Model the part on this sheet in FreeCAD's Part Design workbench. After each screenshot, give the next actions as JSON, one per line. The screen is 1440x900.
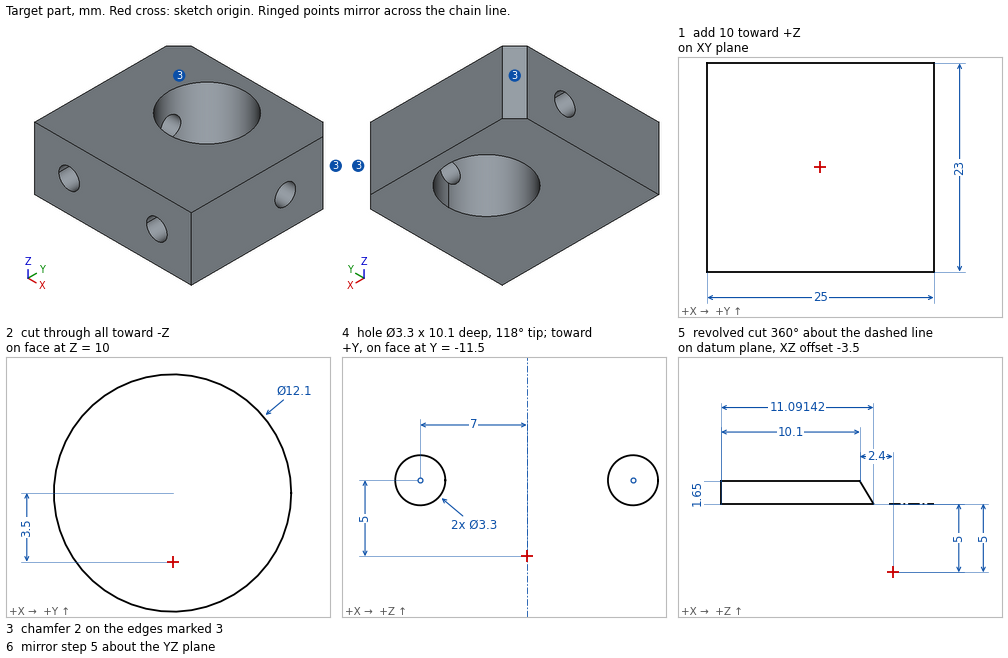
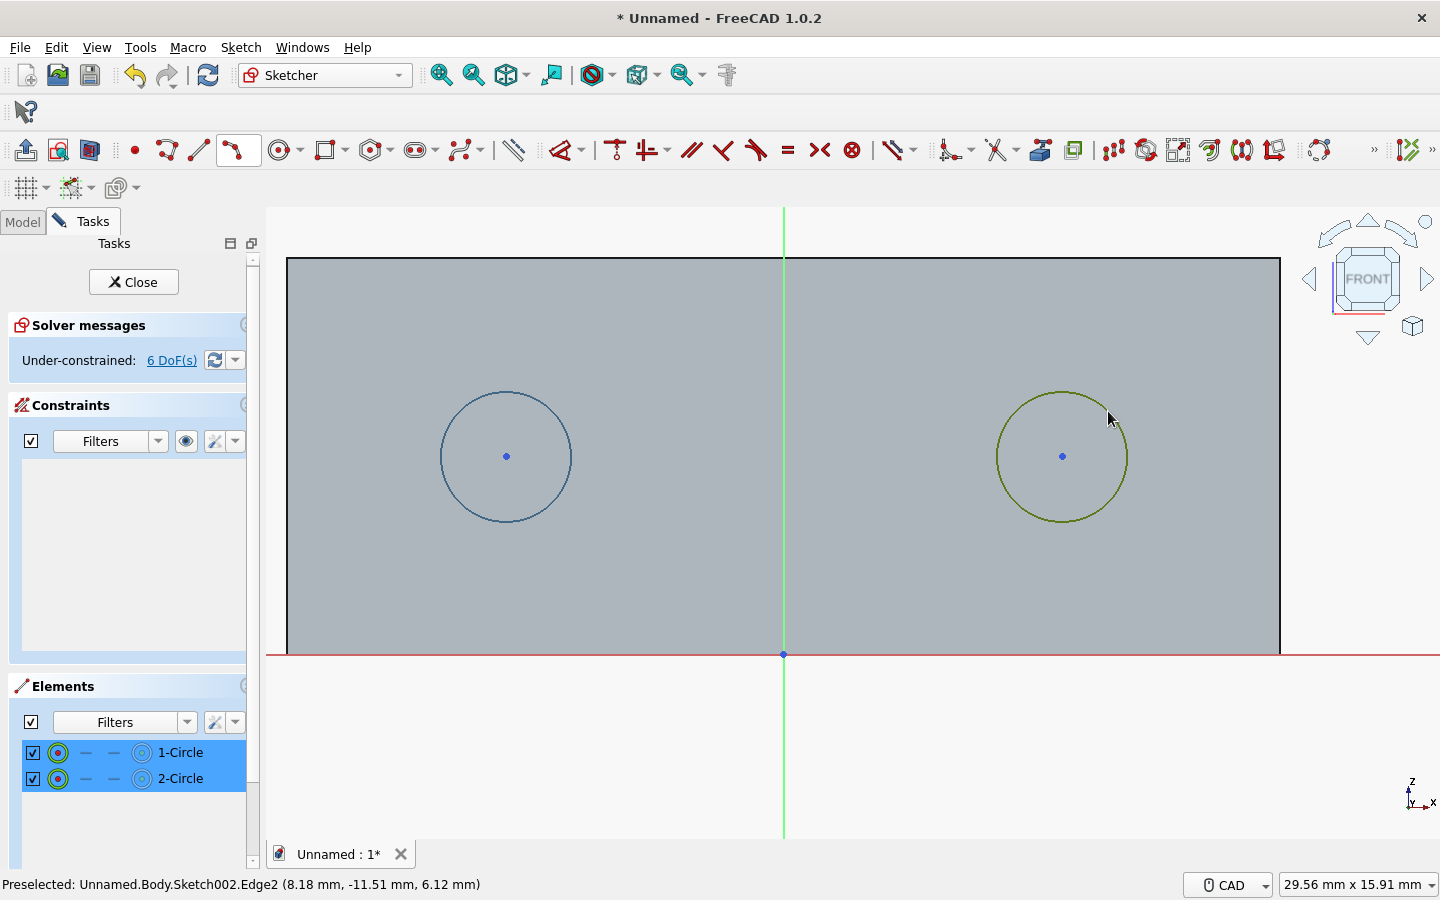
{"action": "left_click", "coordinate": [788, 150]}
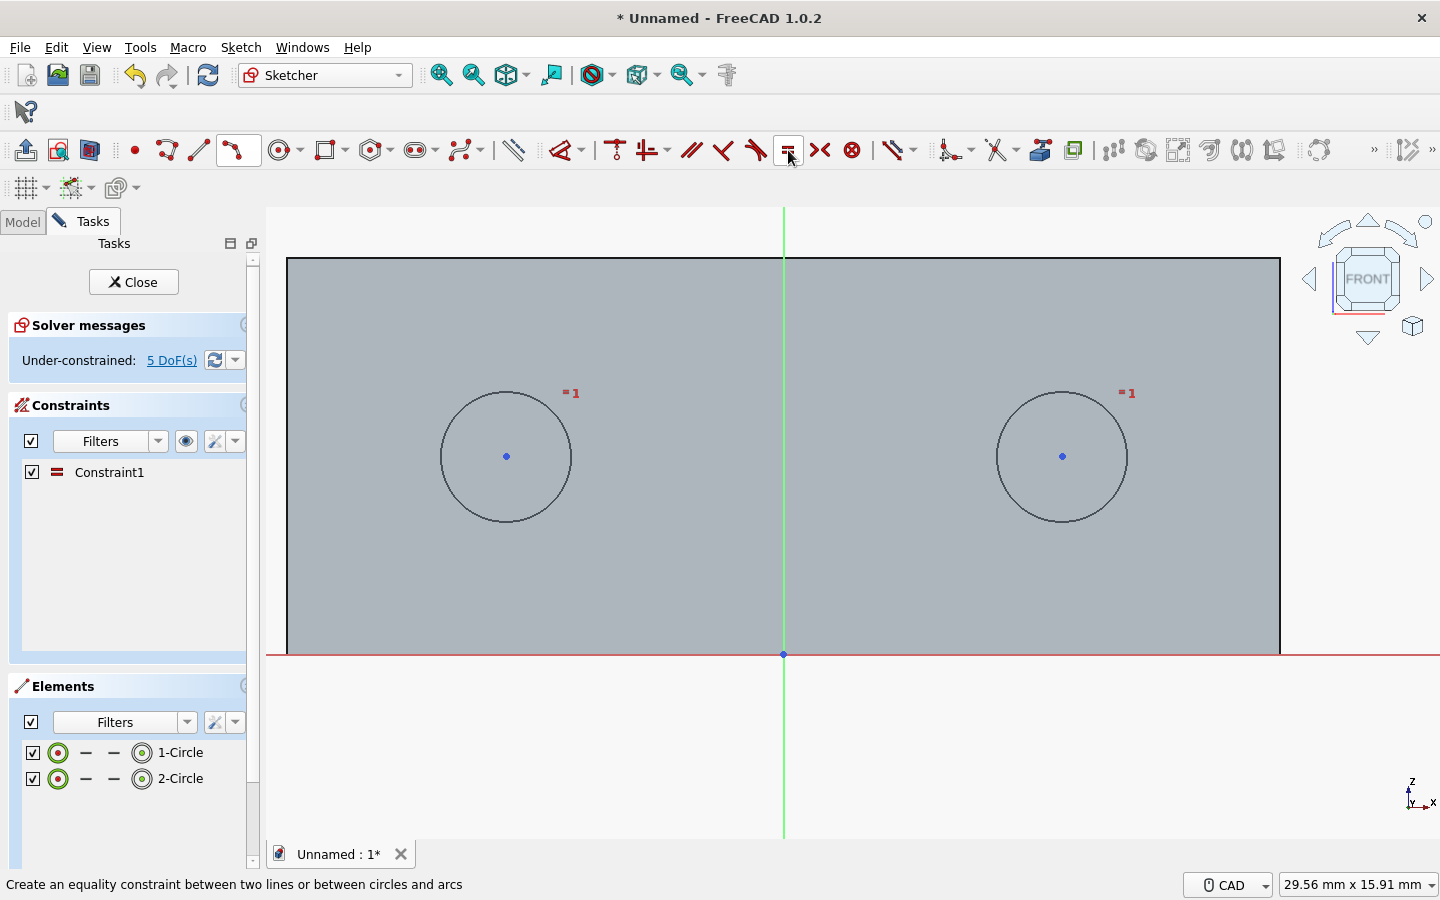
{"action": "left_click", "coordinate": [506, 457]}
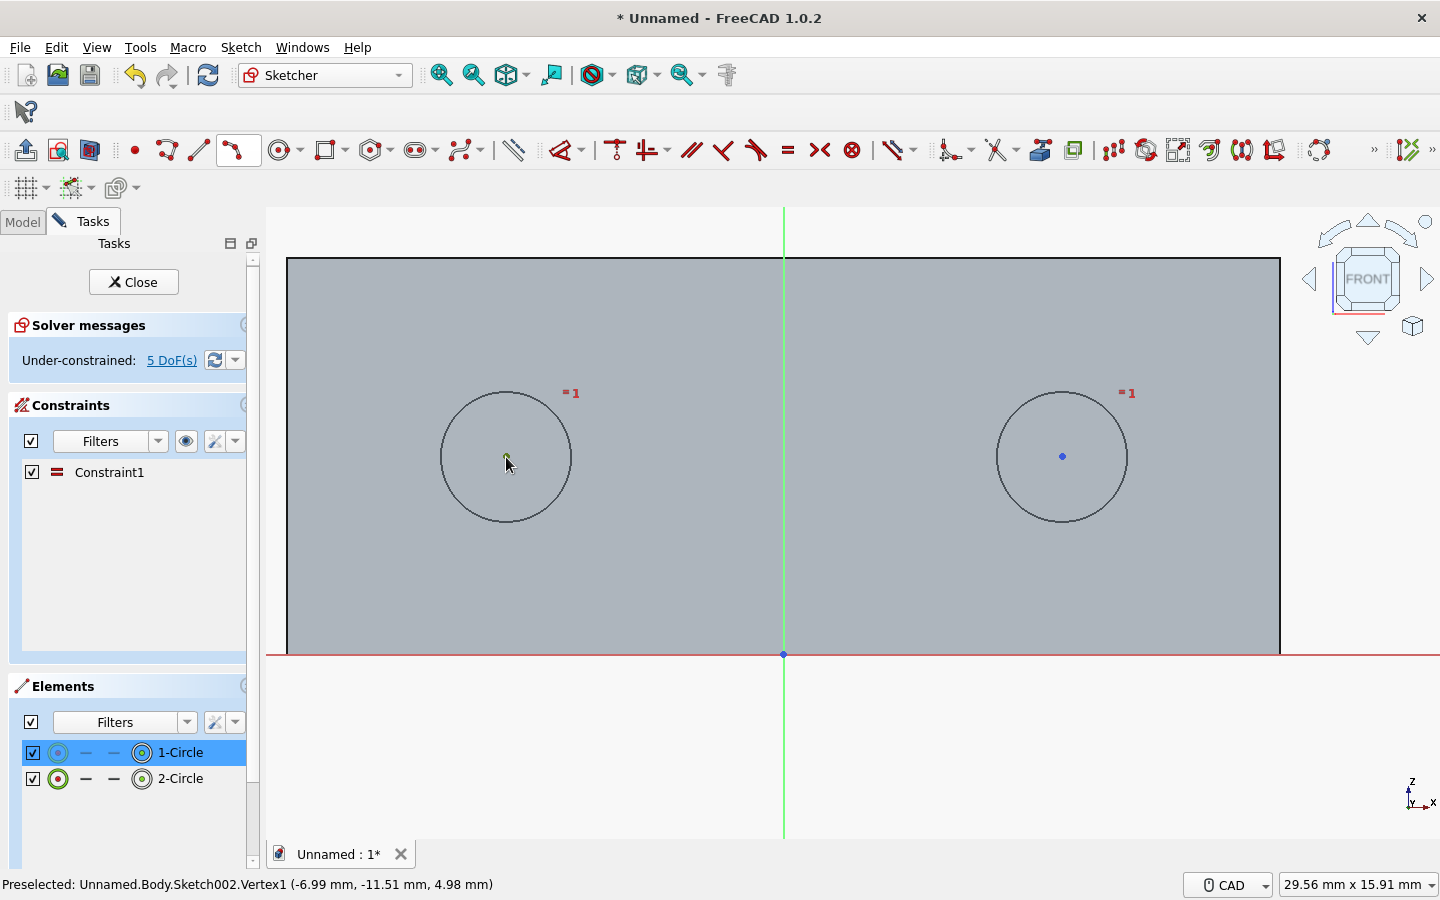
{"action": "left_click", "coordinate": [1062, 457]}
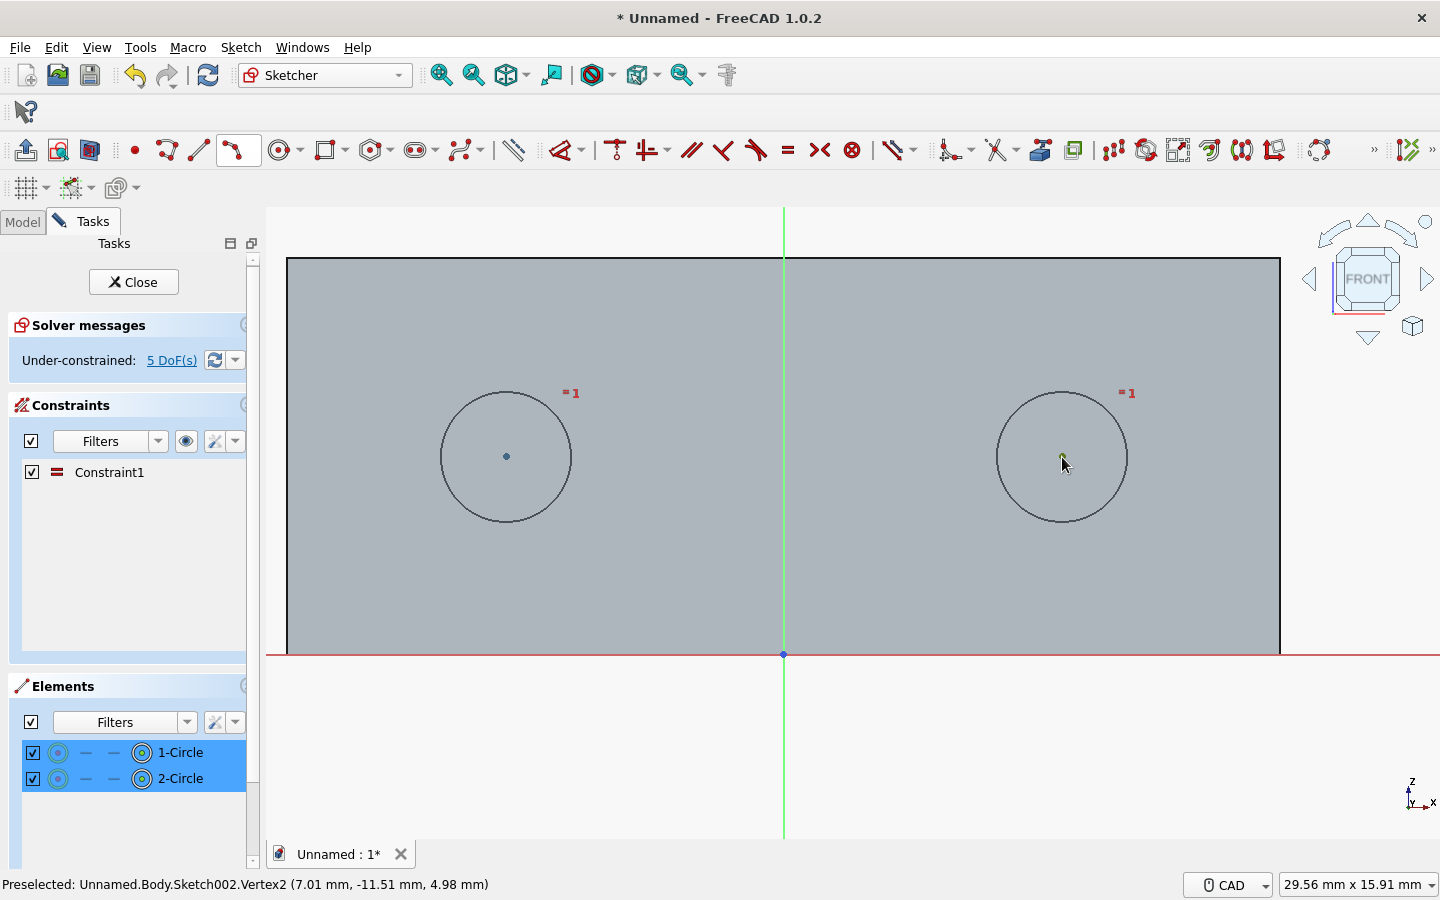
{"action": "left_click", "coordinate": [784, 770]}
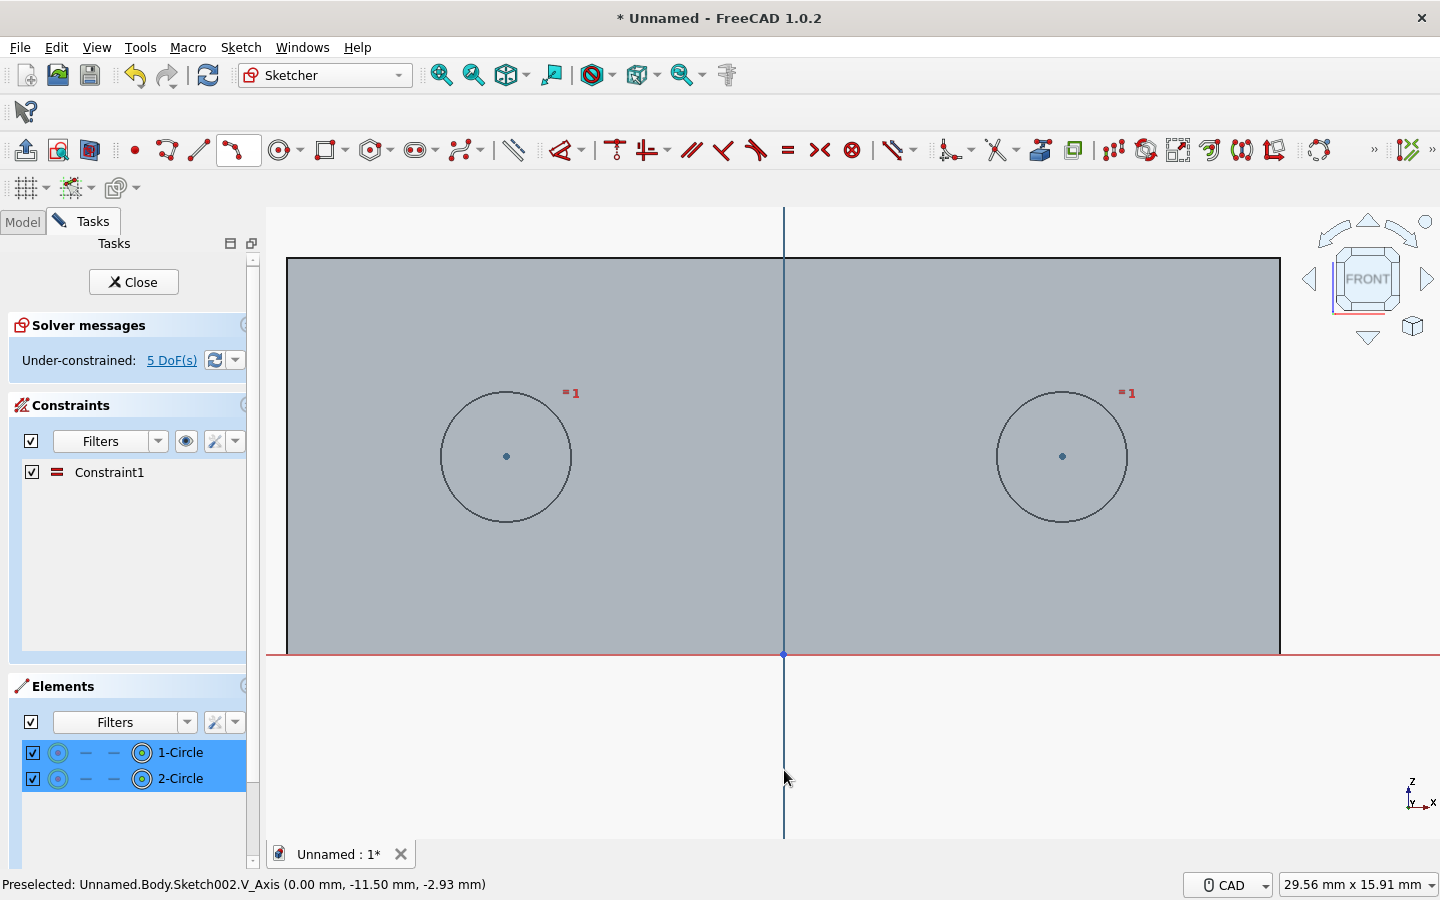
{"action": "key", "text": "s"}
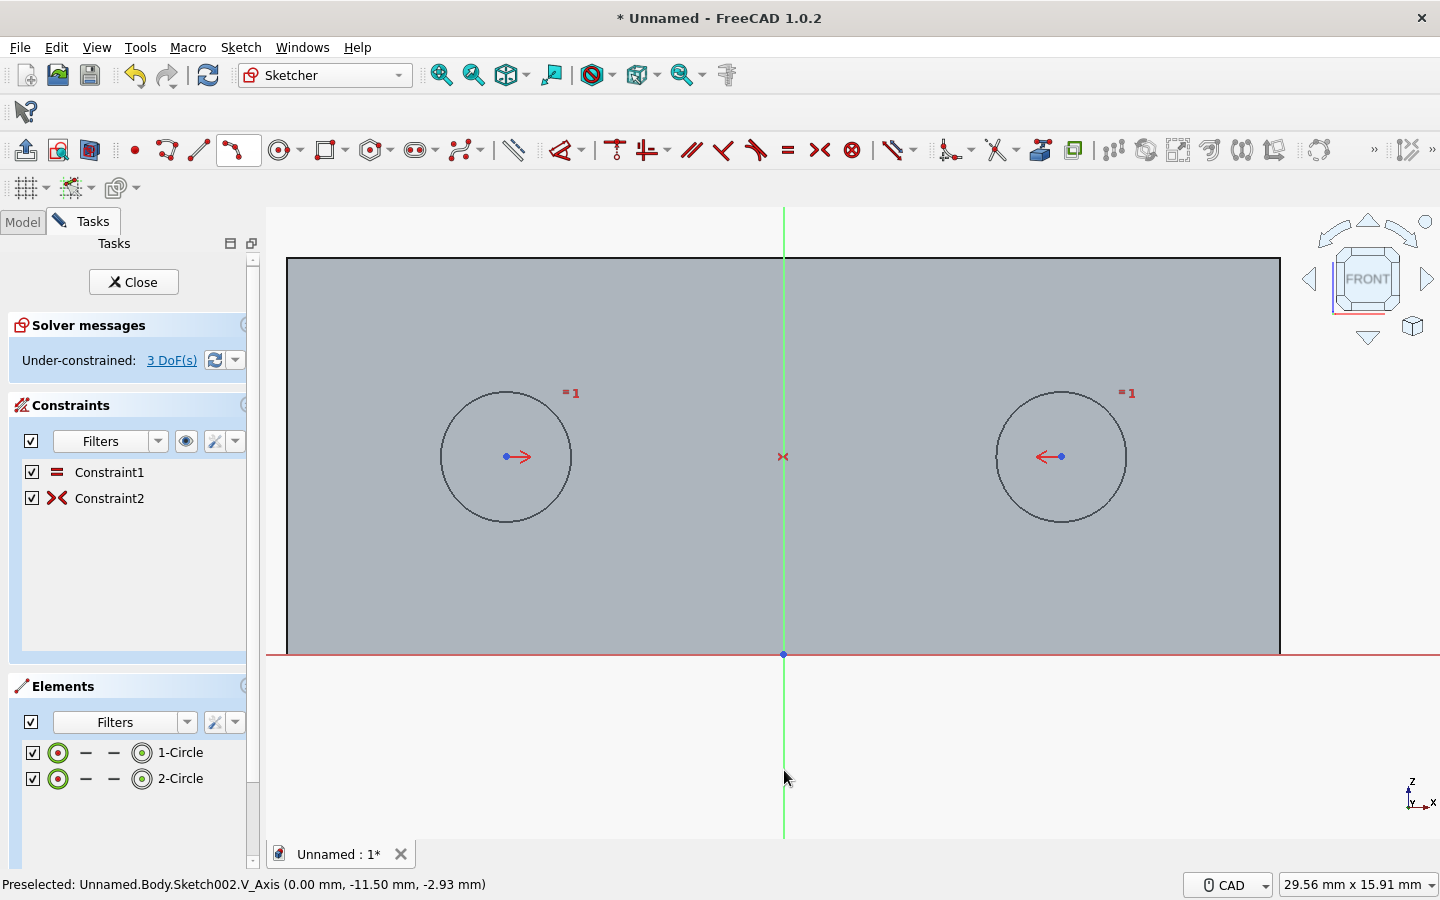
{"action": "key", "text": "d"}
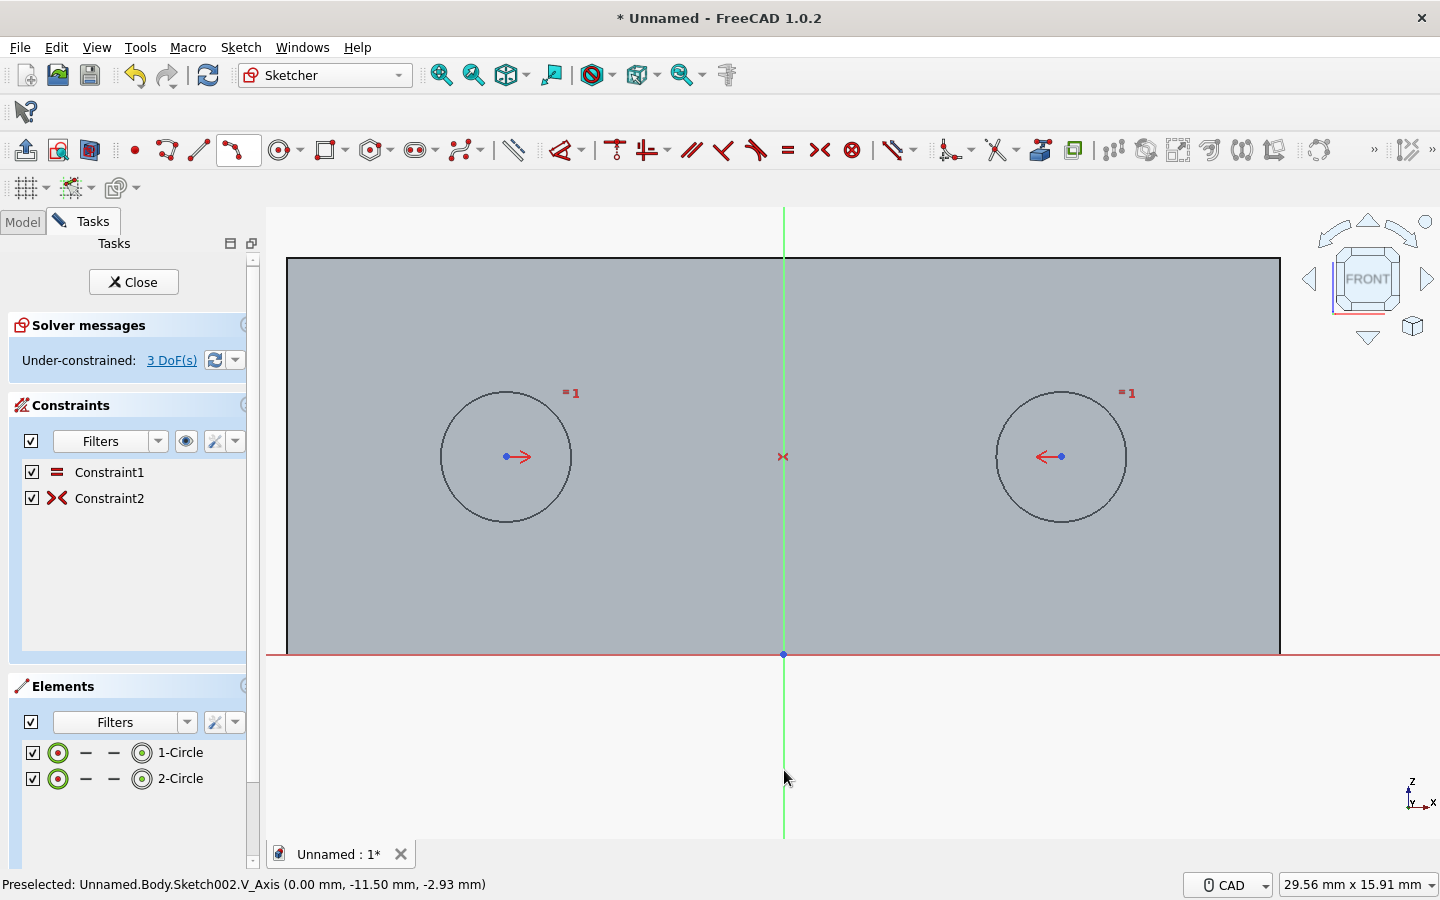
{"action": "left_click", "coordinate": [552, 411]}
{"action": "left_click", "coordinate": [575, 388]}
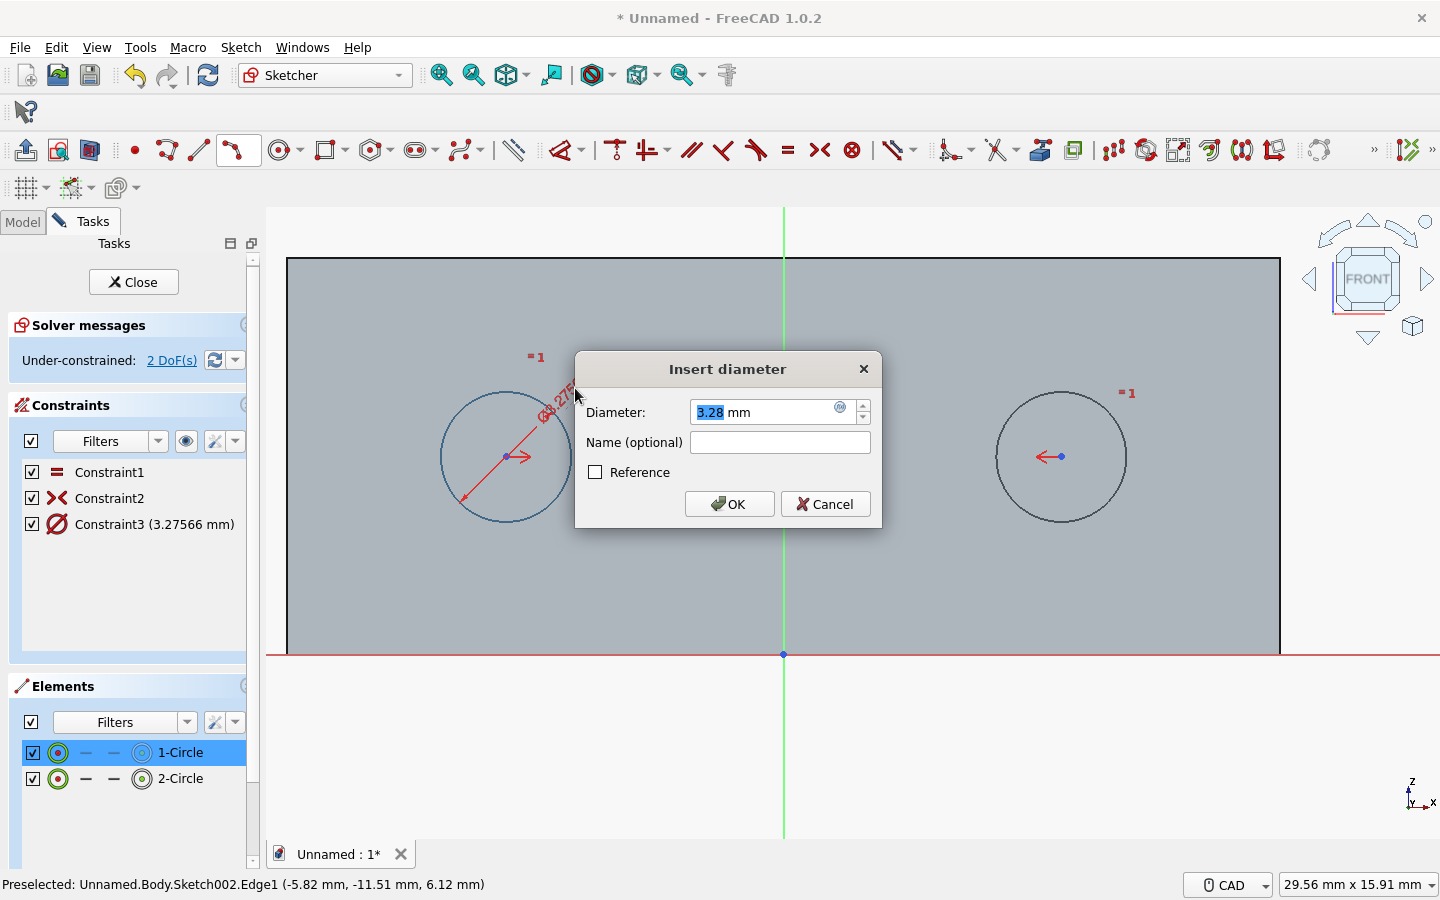
{"action": "type", "text": "3.3"}
{"action": "key", "text": "Return"}